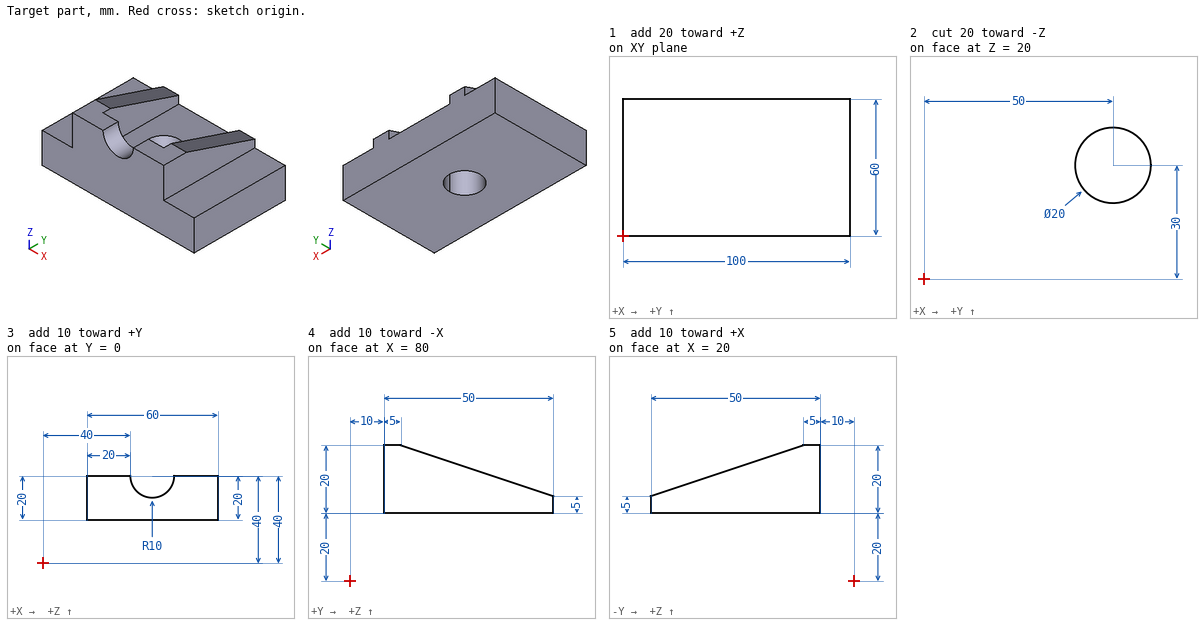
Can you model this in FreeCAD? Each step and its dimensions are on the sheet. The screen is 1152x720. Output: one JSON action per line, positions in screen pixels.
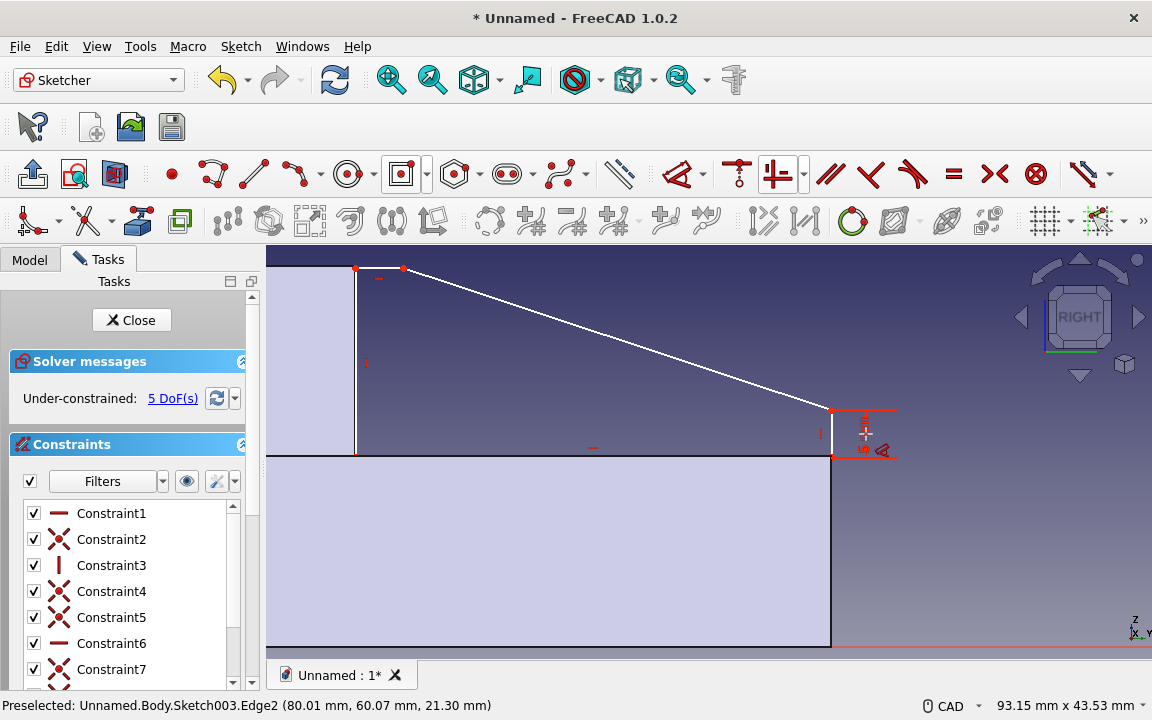
{"action": "scroll", "coordinate": [833, 443], "scroll_direction": "down", "scroll_amount": 2}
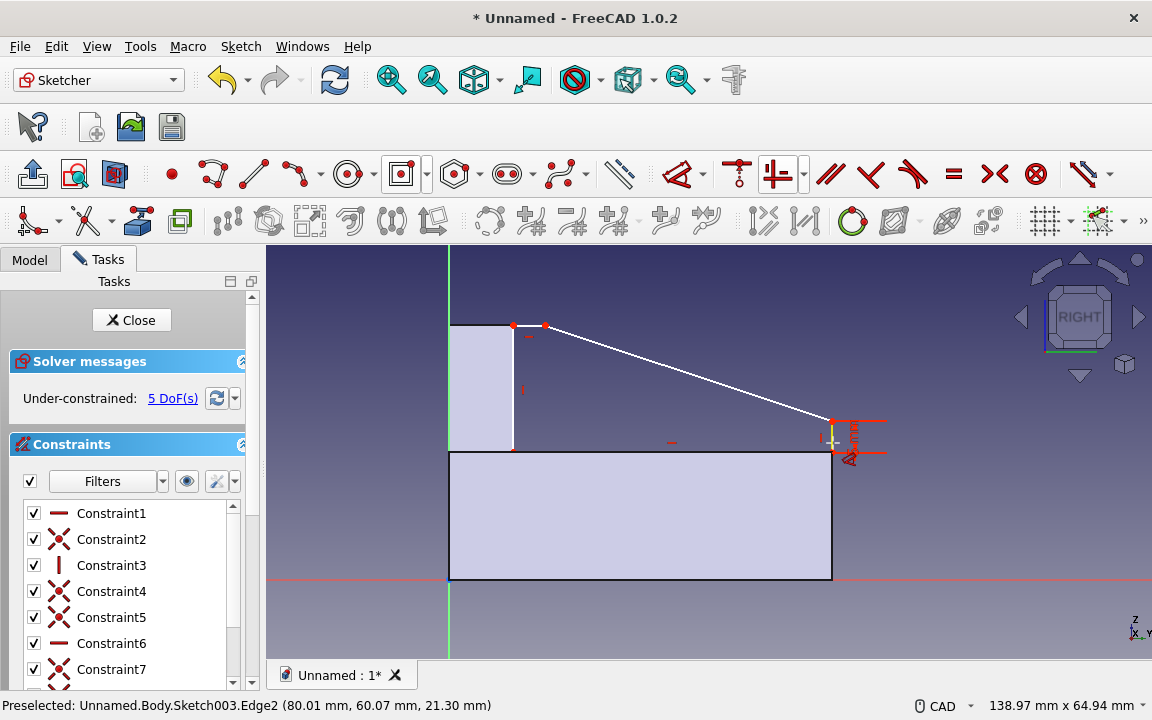
{"action": "scroll", "coordinate": [536, 326], "scroll_direction": "up", "scroll_amount": 2}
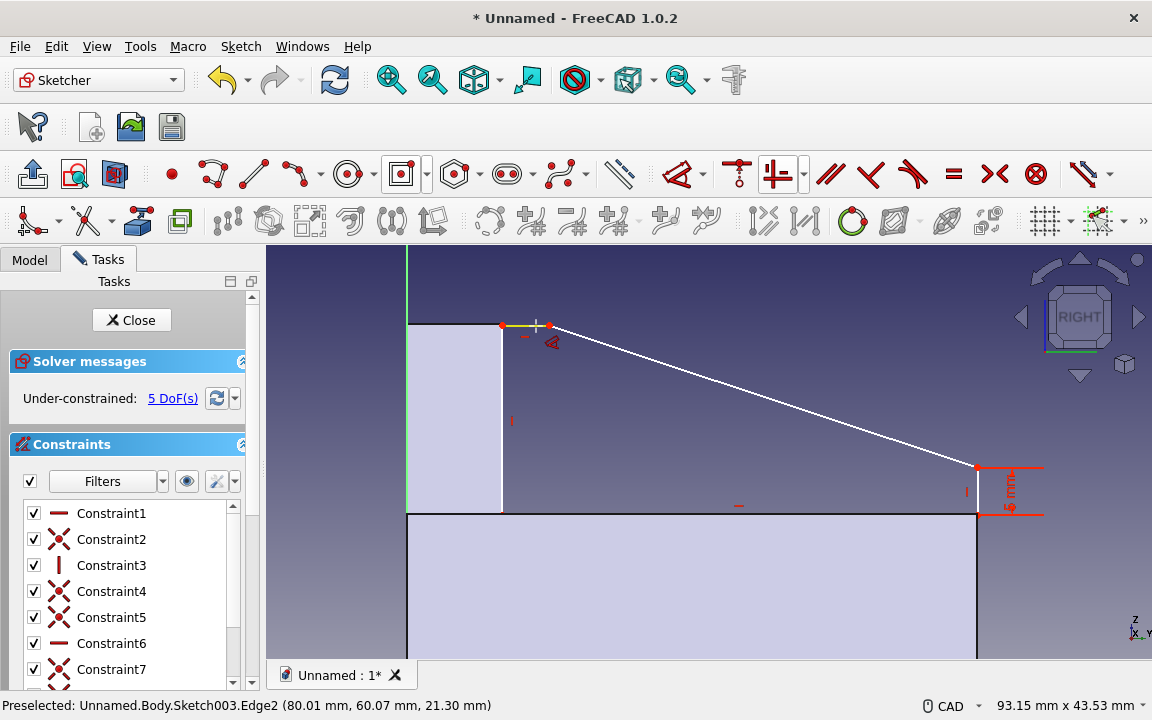
{"action": "left_click", "coordinate": [535, 326]}
{"action": "left_click", "coordinate": [526, 292]}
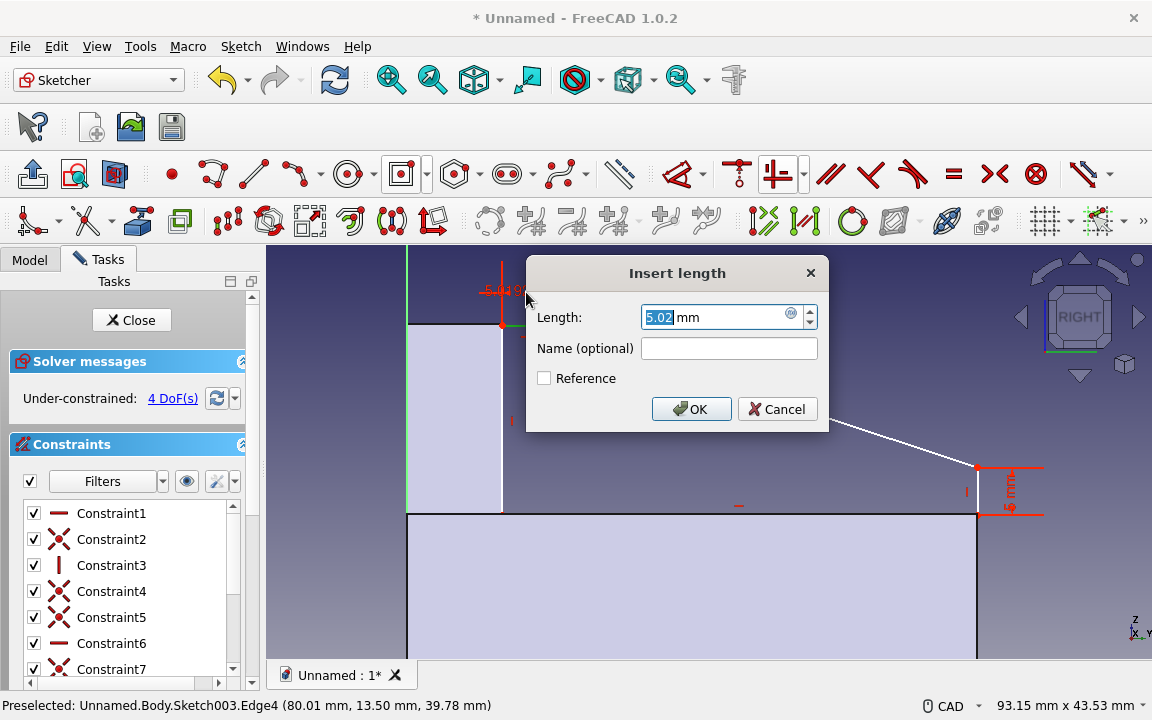
{"action": "type", "text": "5"}
{"action": "key", "text": "Return"}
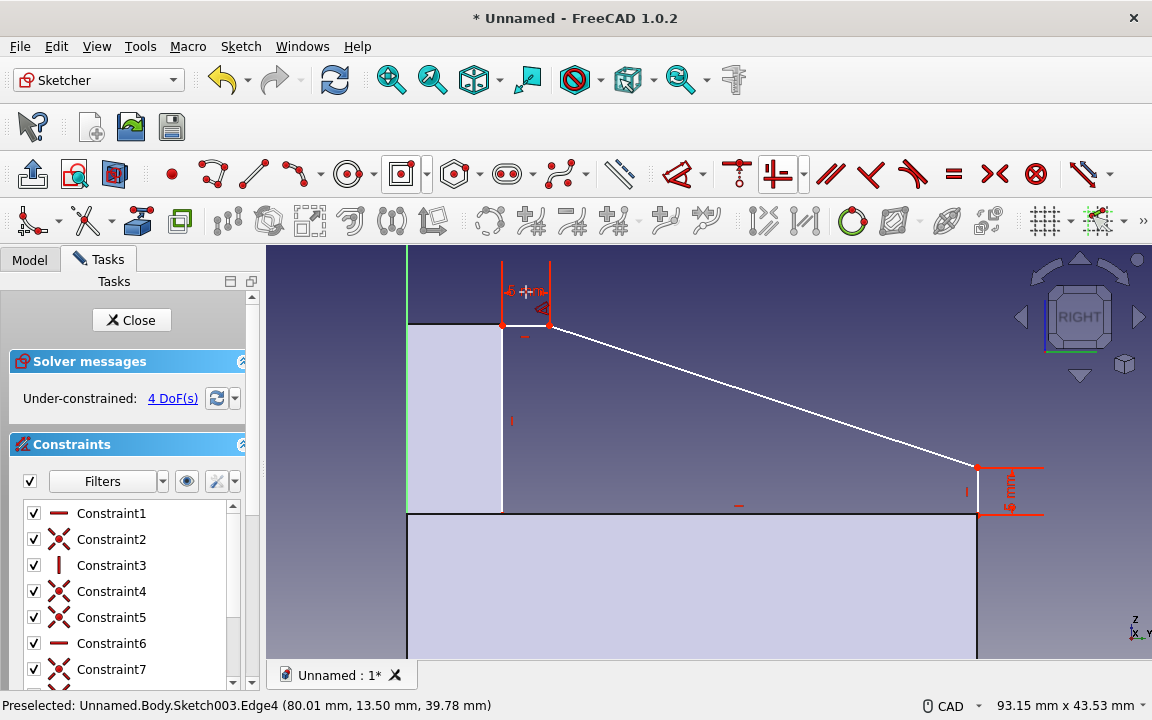
{"action": "left_click", "coordinate": [645, 515]}
{"action": "left_click", "coordinate": [740, 549]}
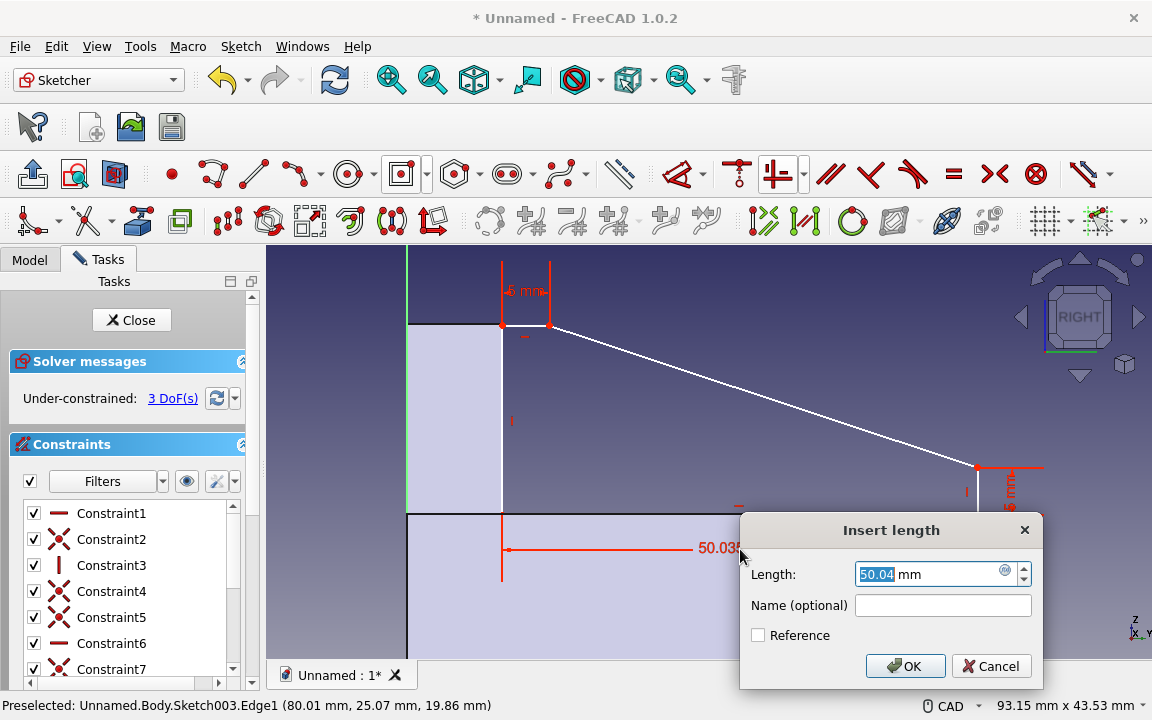
{"action": "type", "text": "50"}
{"action": "key", "text": "Return"}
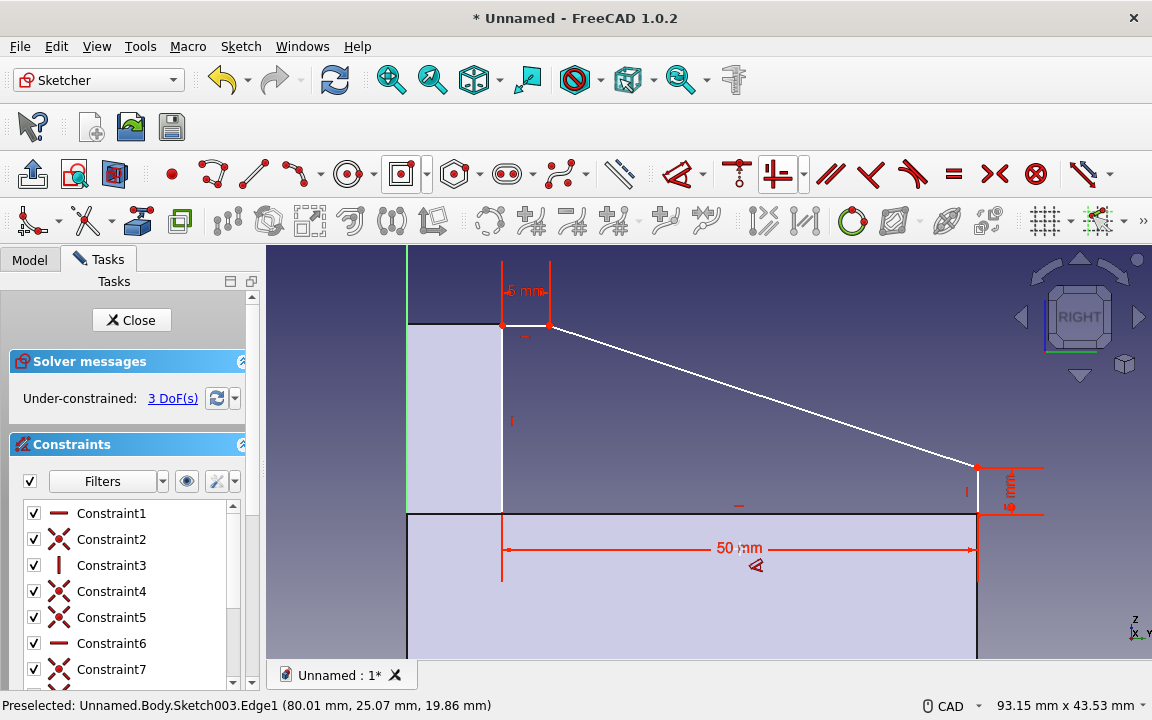
{"action": "left_click", "coordinate": [502, 383]}
{"action": "left_click", "coordinate": [468, 421]}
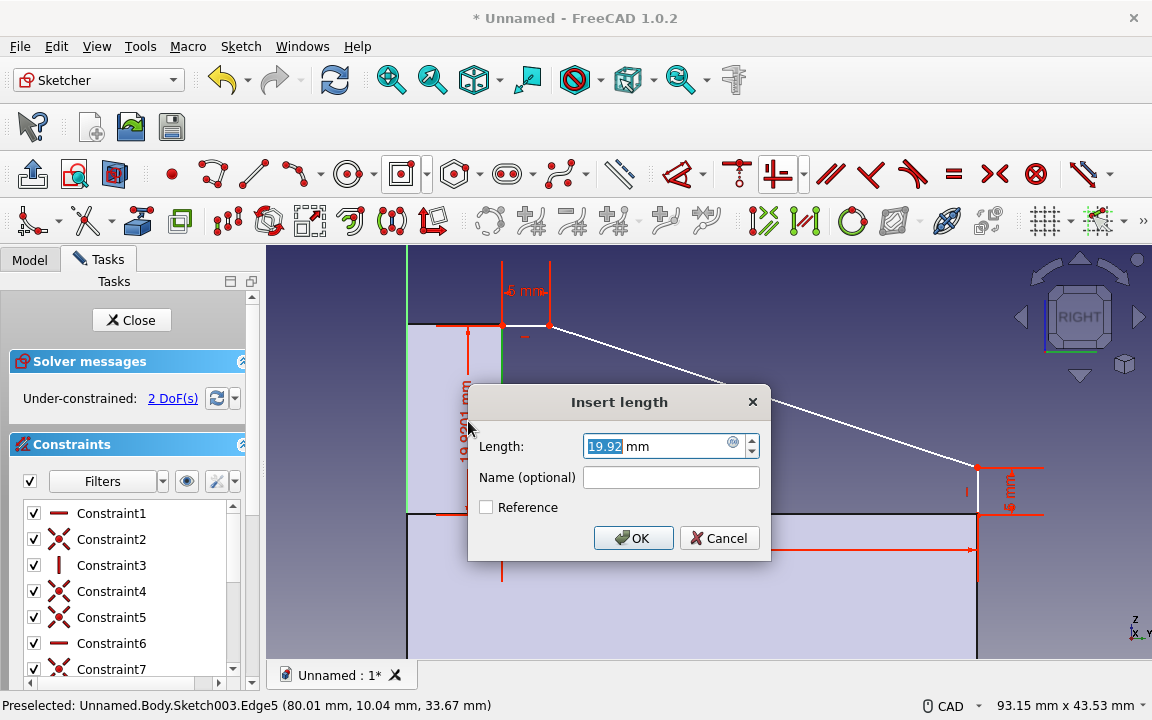
{"action": "type", "text": "20"}
{"action": "key", "text": "Return"}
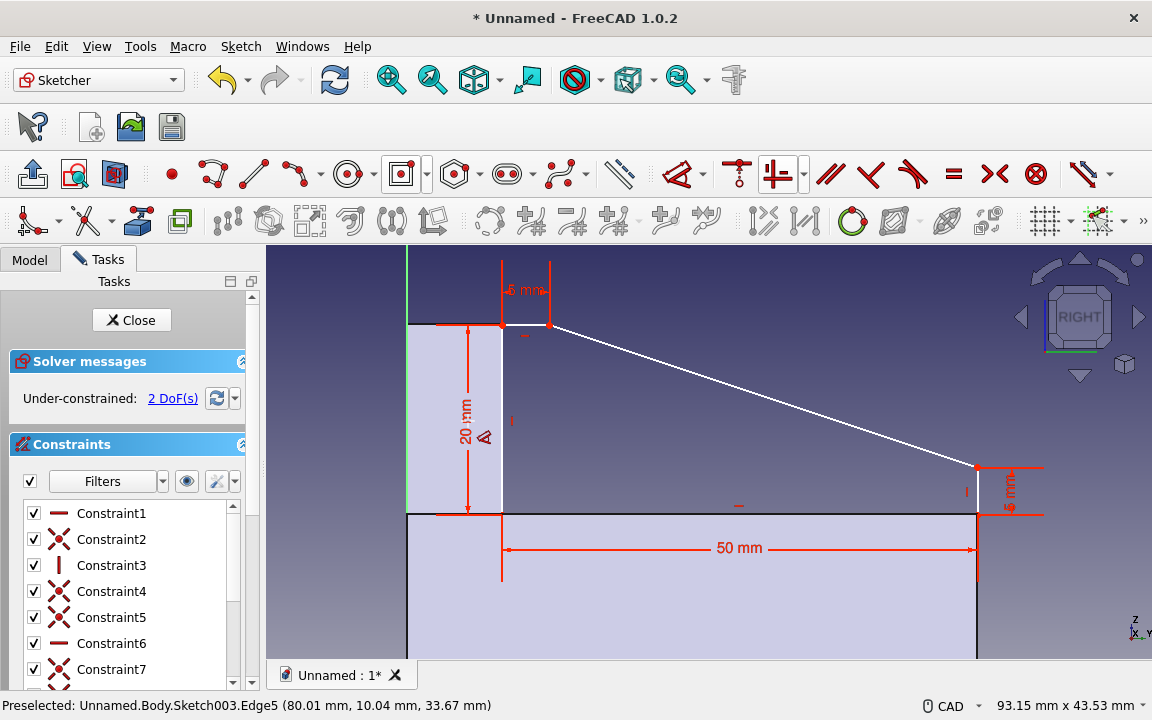
{"action": "left_click", "coordinate": [502, 515]}
{"action": "left_click", "coordinate": [454, 481]}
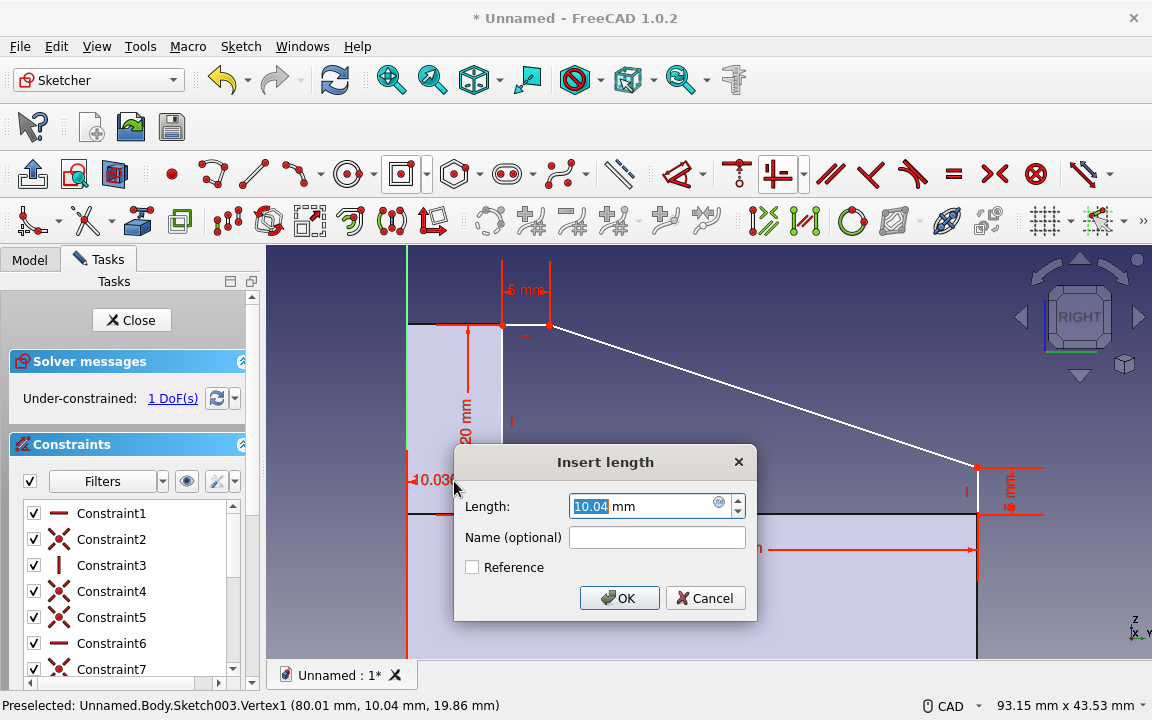
{"action": "type", "text": "10"}
{"action": "key", "text": "Return"}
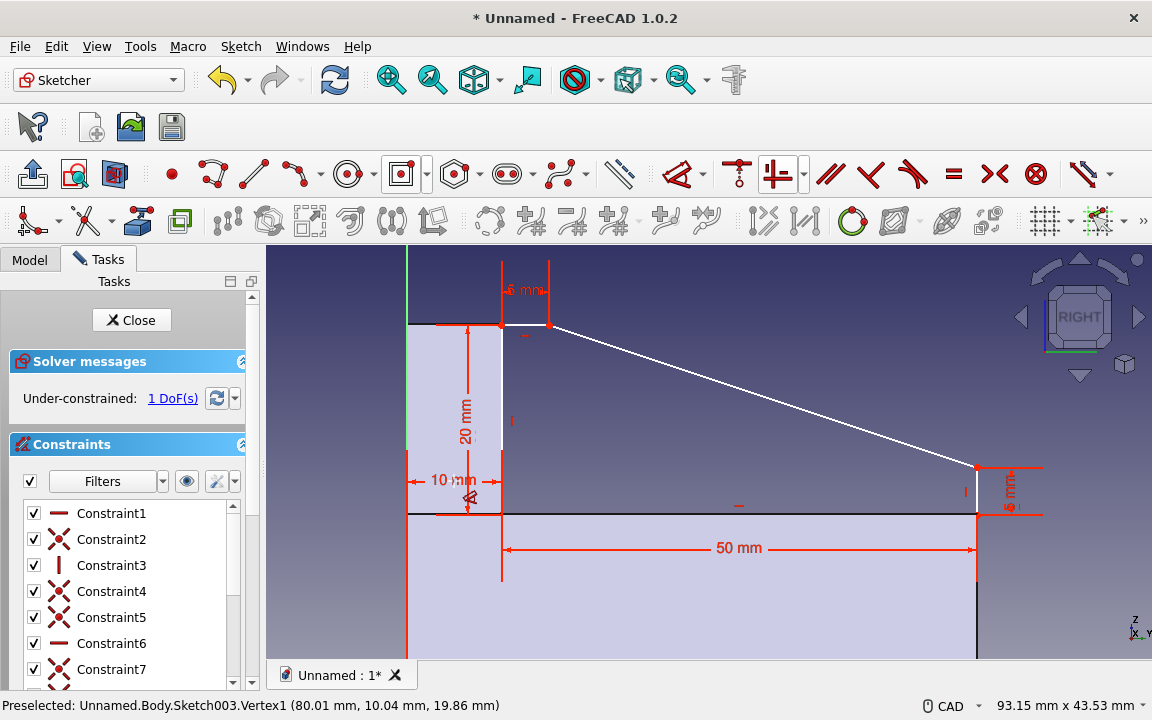
{"action": "left_click", "coordinate": [502, 515]}
{"action": "left_click", "coordinate": [373, 573]}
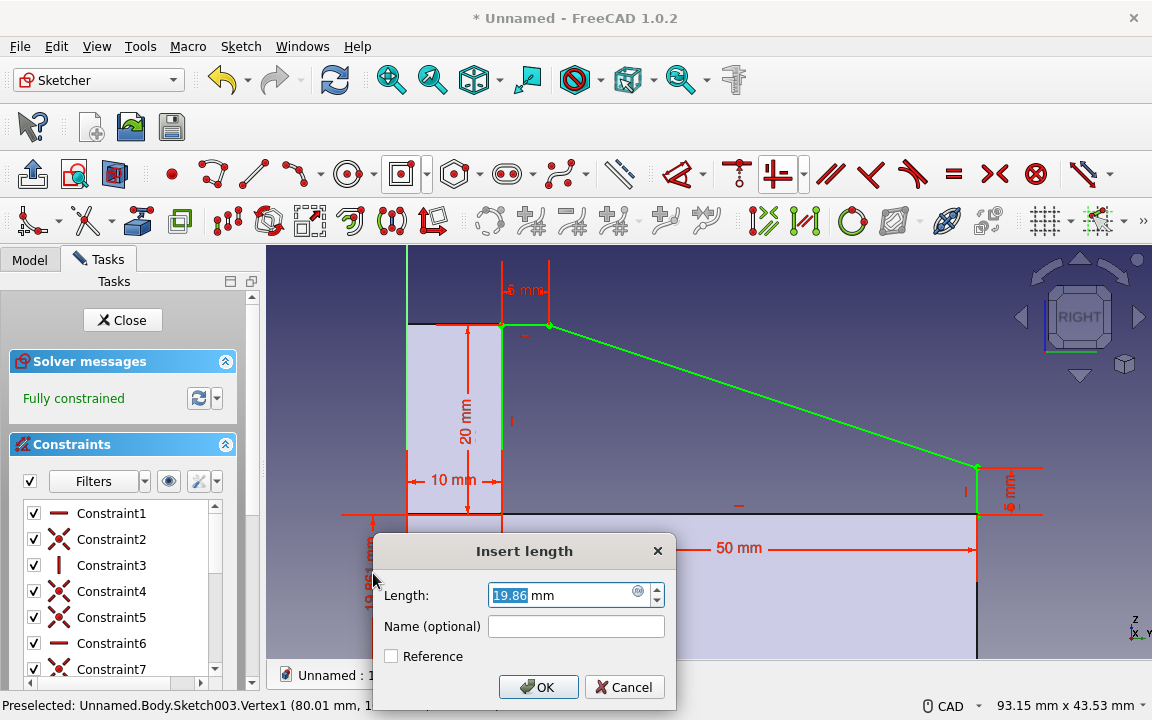
{"action": "type", "text": "20"}
{"action": "key", "text": "Return"}
{"action": "key", "text": "Escape"}